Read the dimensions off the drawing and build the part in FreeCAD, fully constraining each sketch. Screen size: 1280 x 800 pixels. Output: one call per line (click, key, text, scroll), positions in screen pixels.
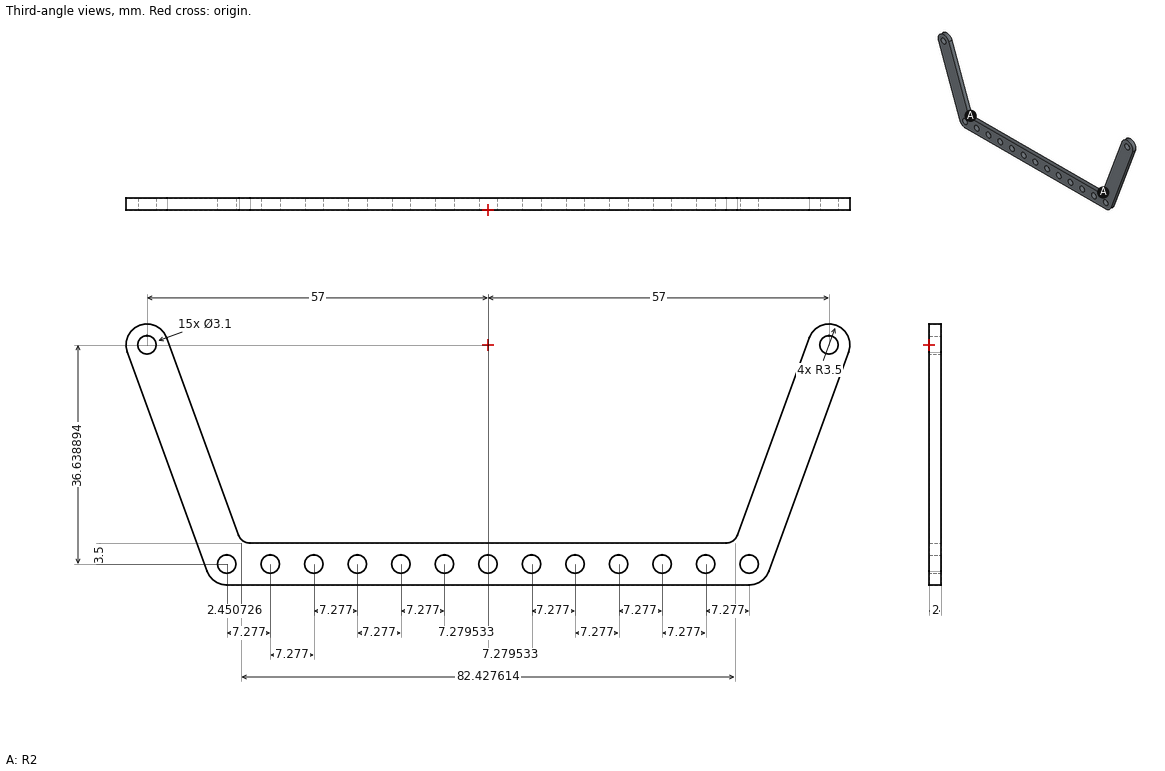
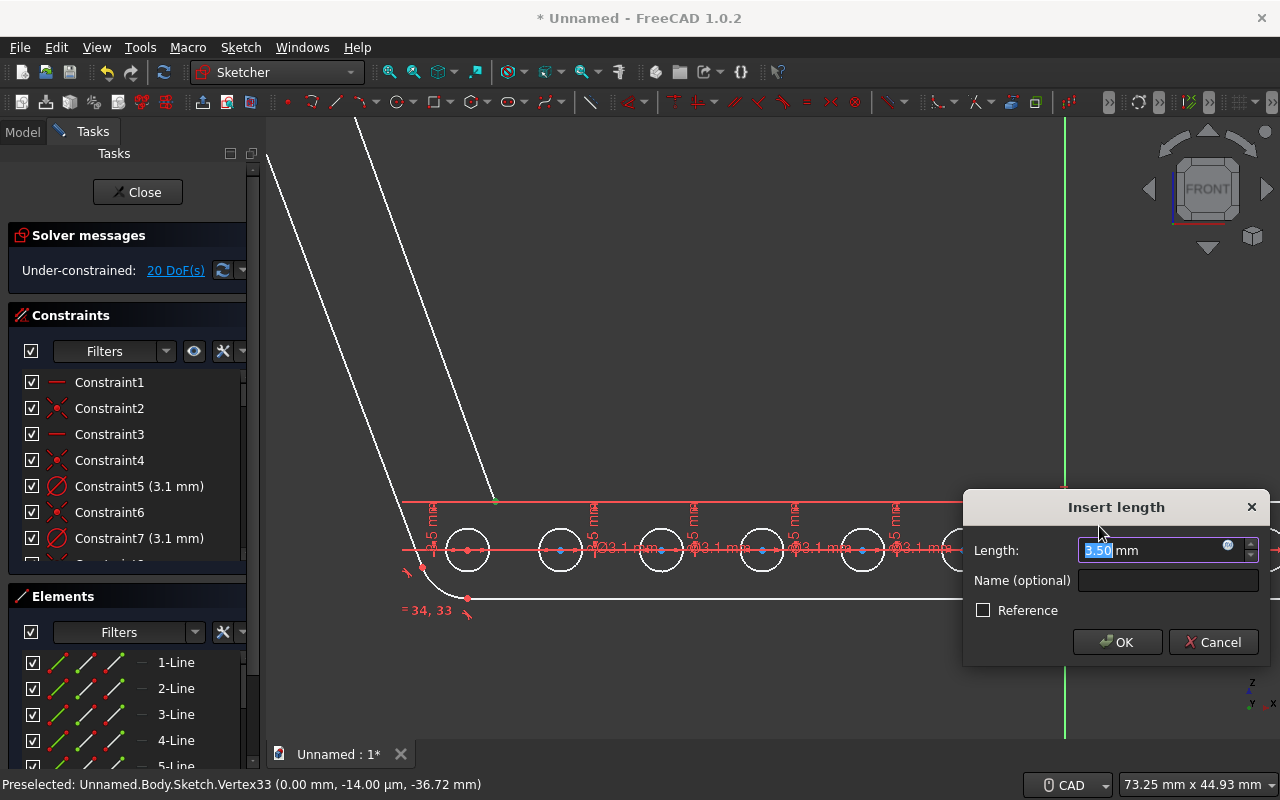
text(3.5)
key(Return)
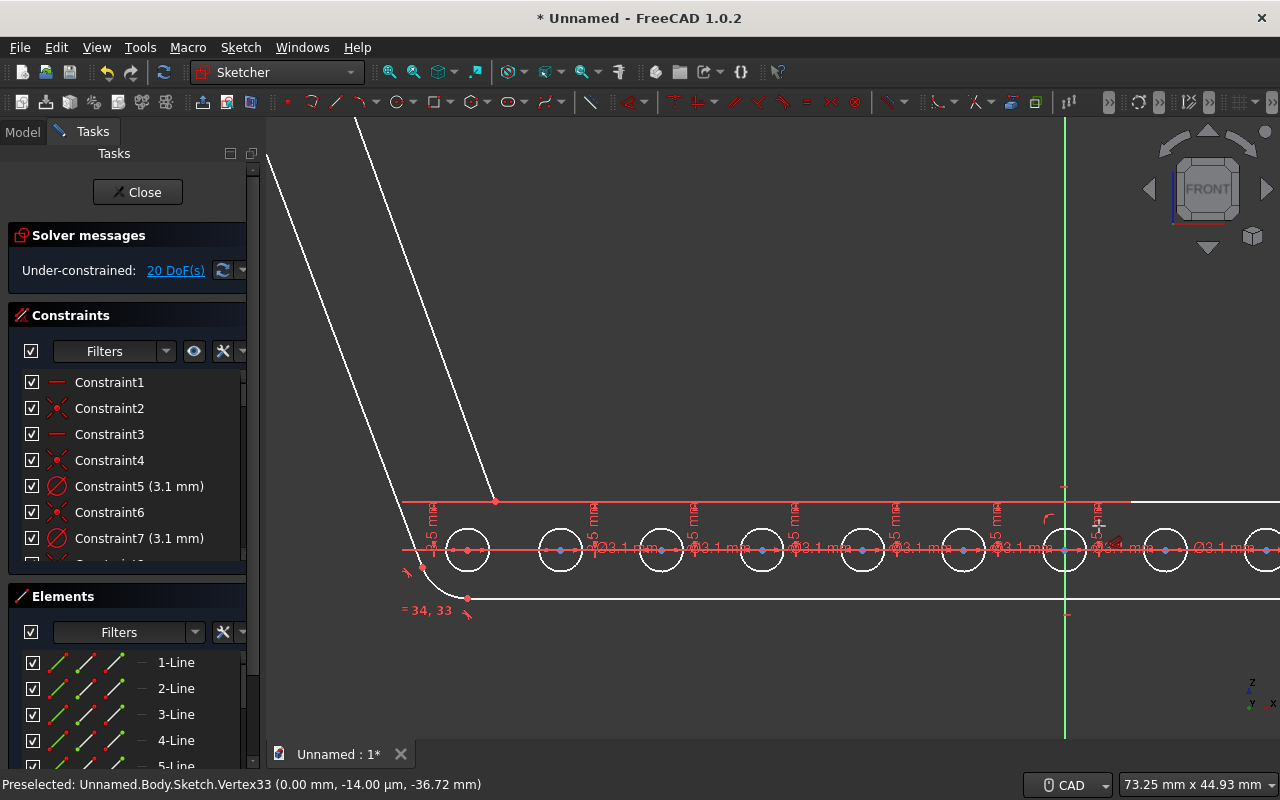
scroll(495, 504, down, 5)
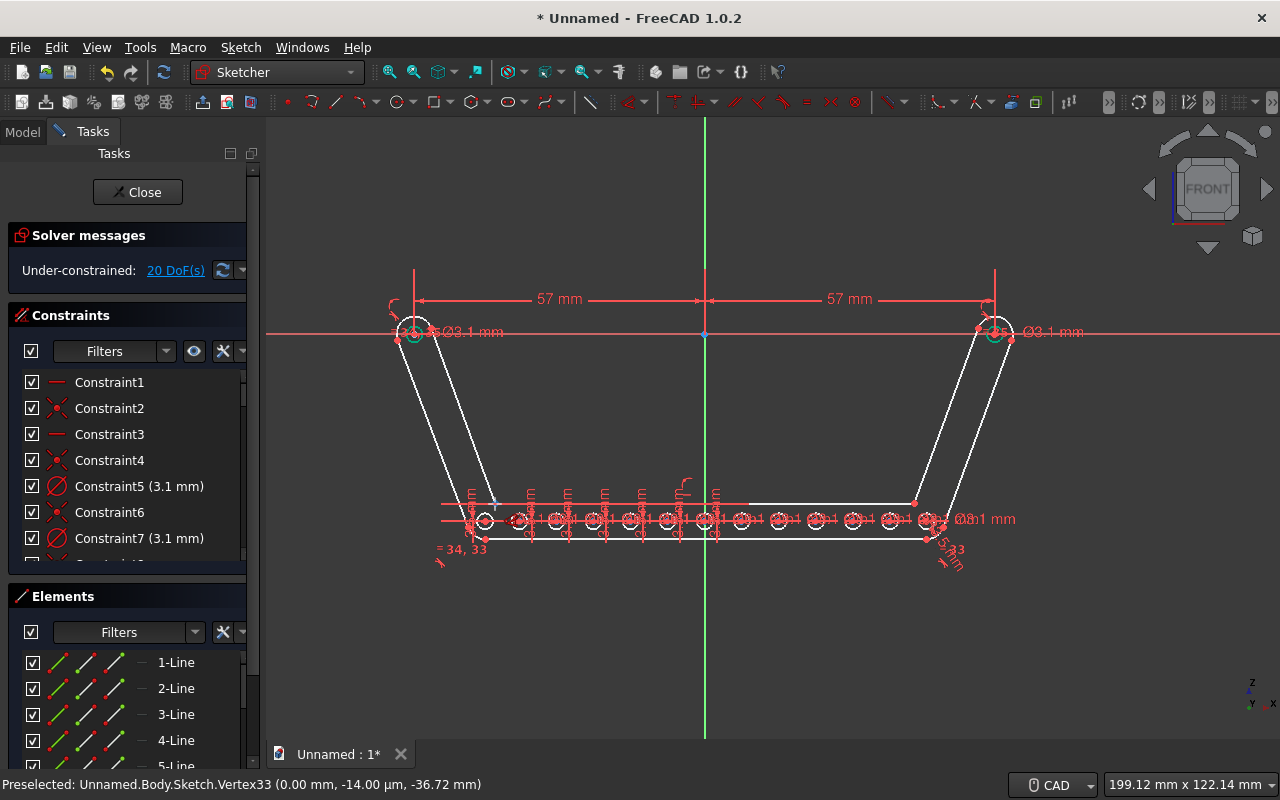
scroll(914, 504, up, 5)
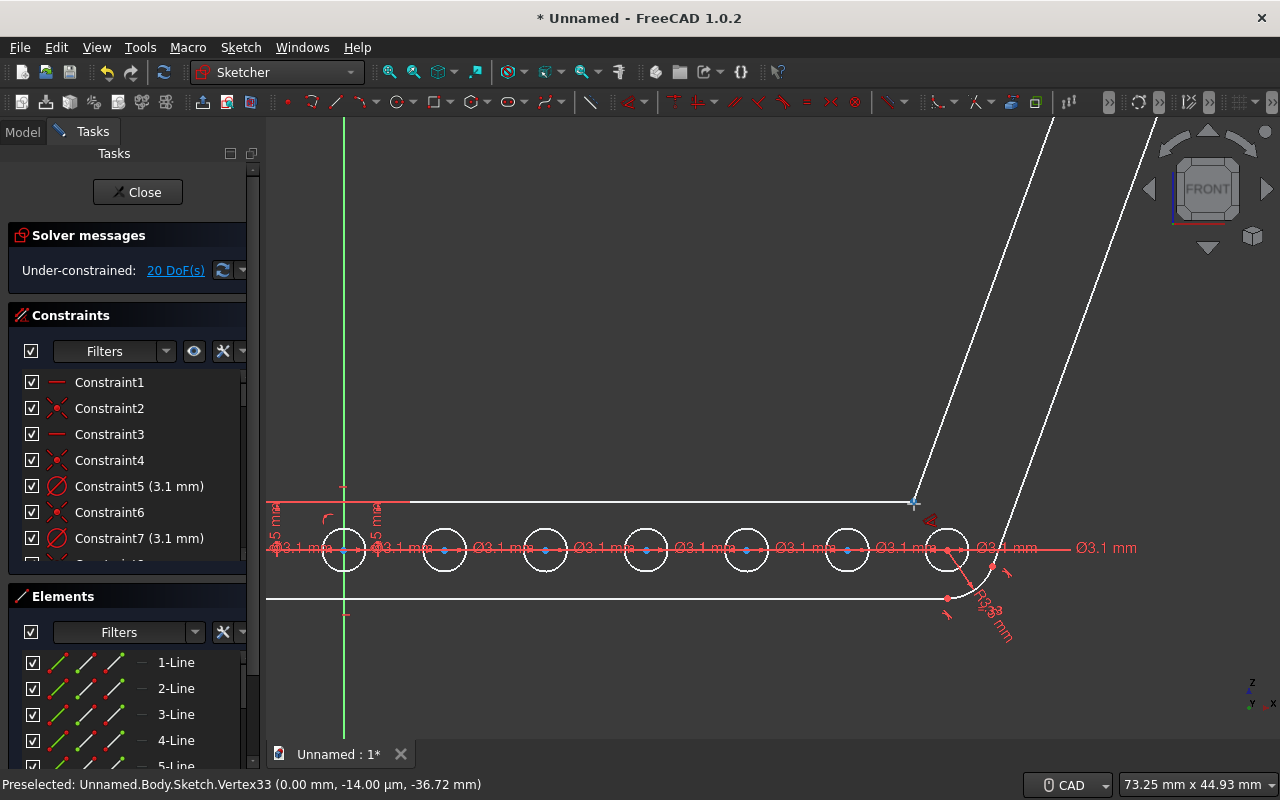
click(913, 502)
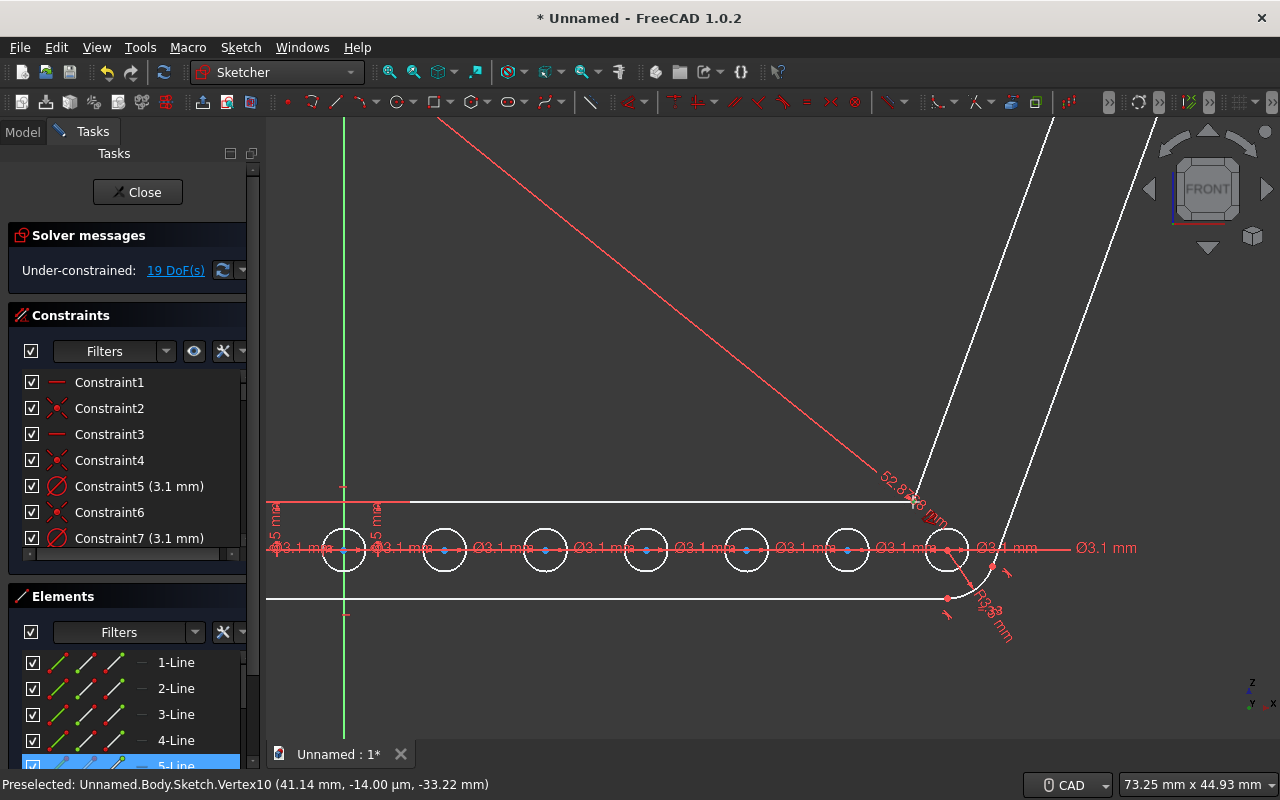
click(445, 550)
click(947, 515)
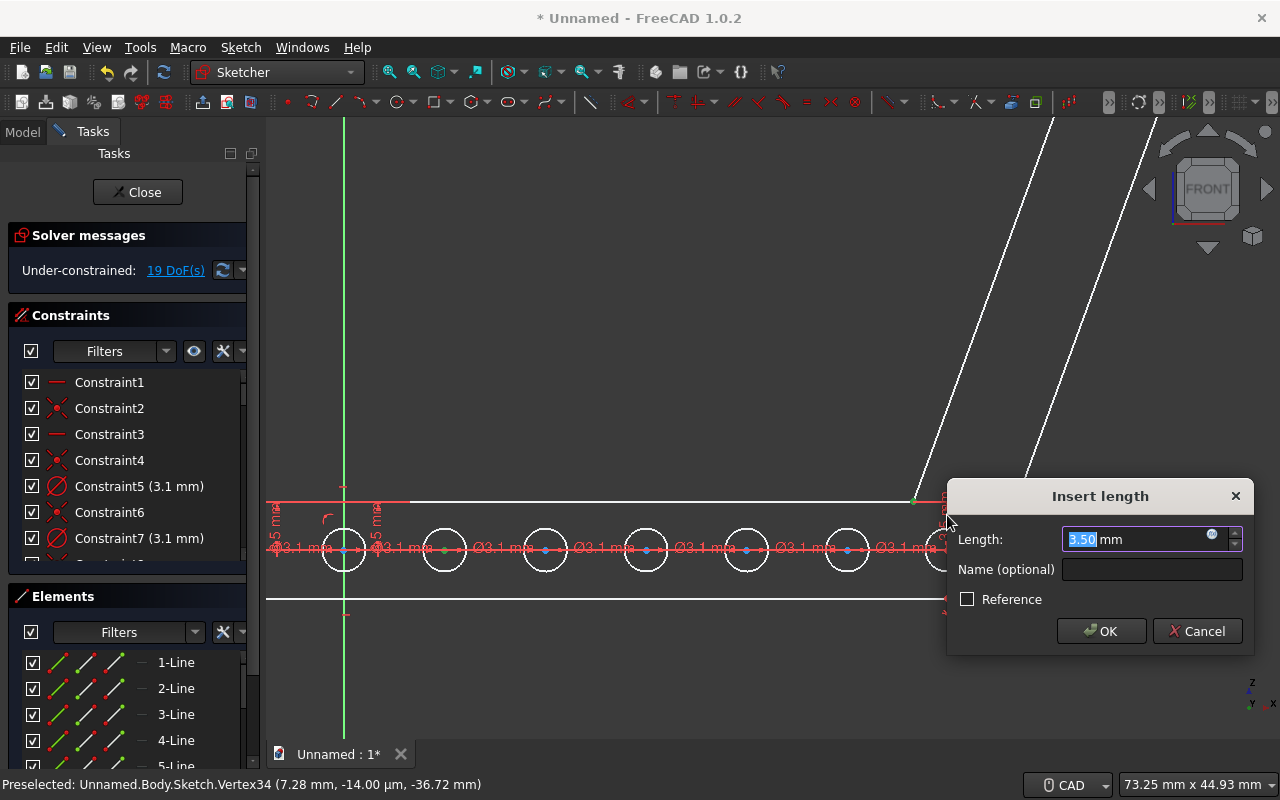
text(3.5)
key(Return)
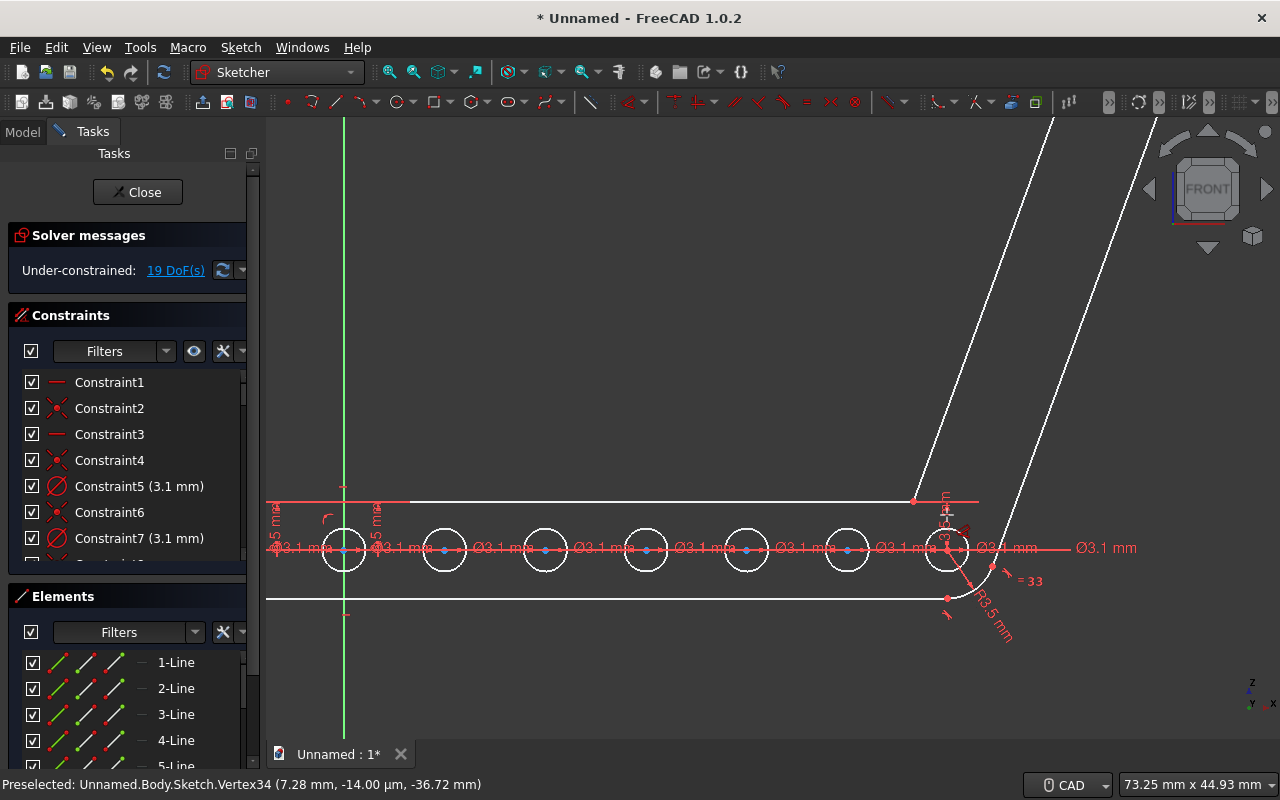
click(913, 502)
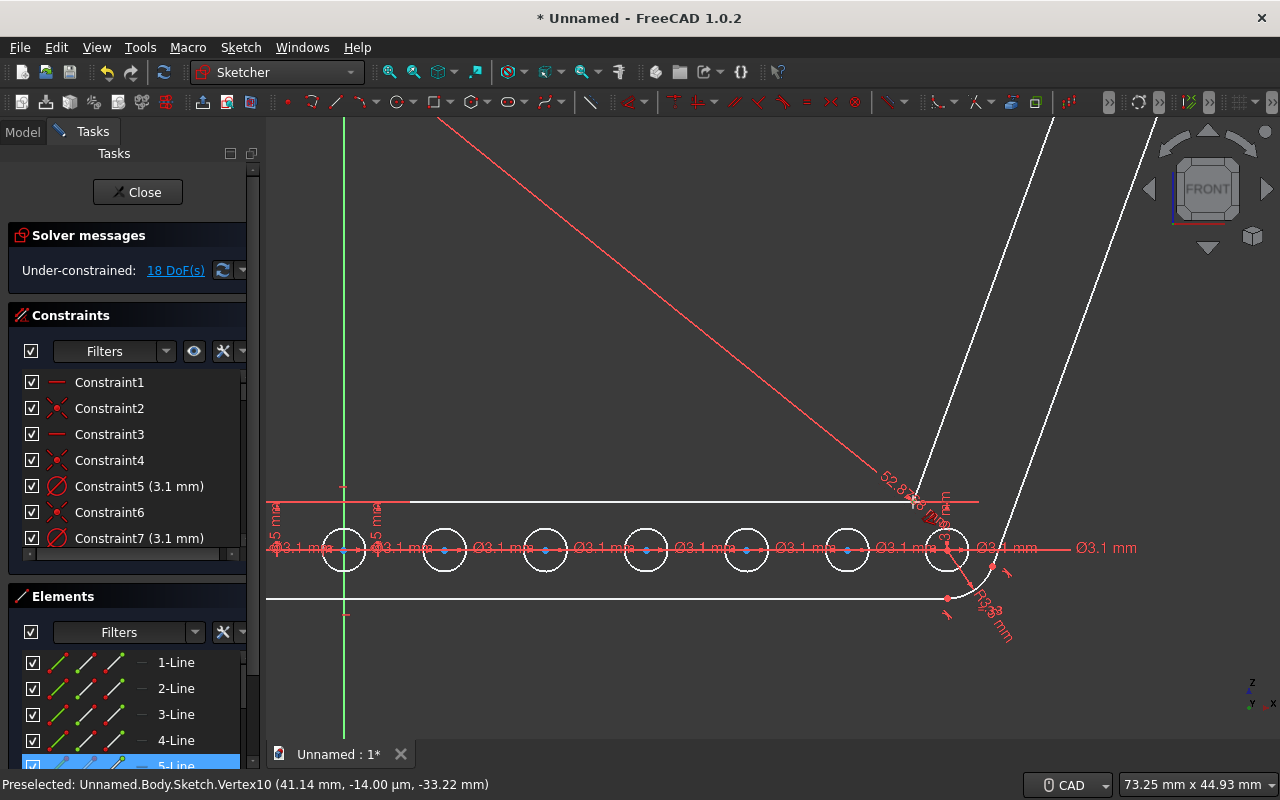
click(545, 550)
click(947, 543)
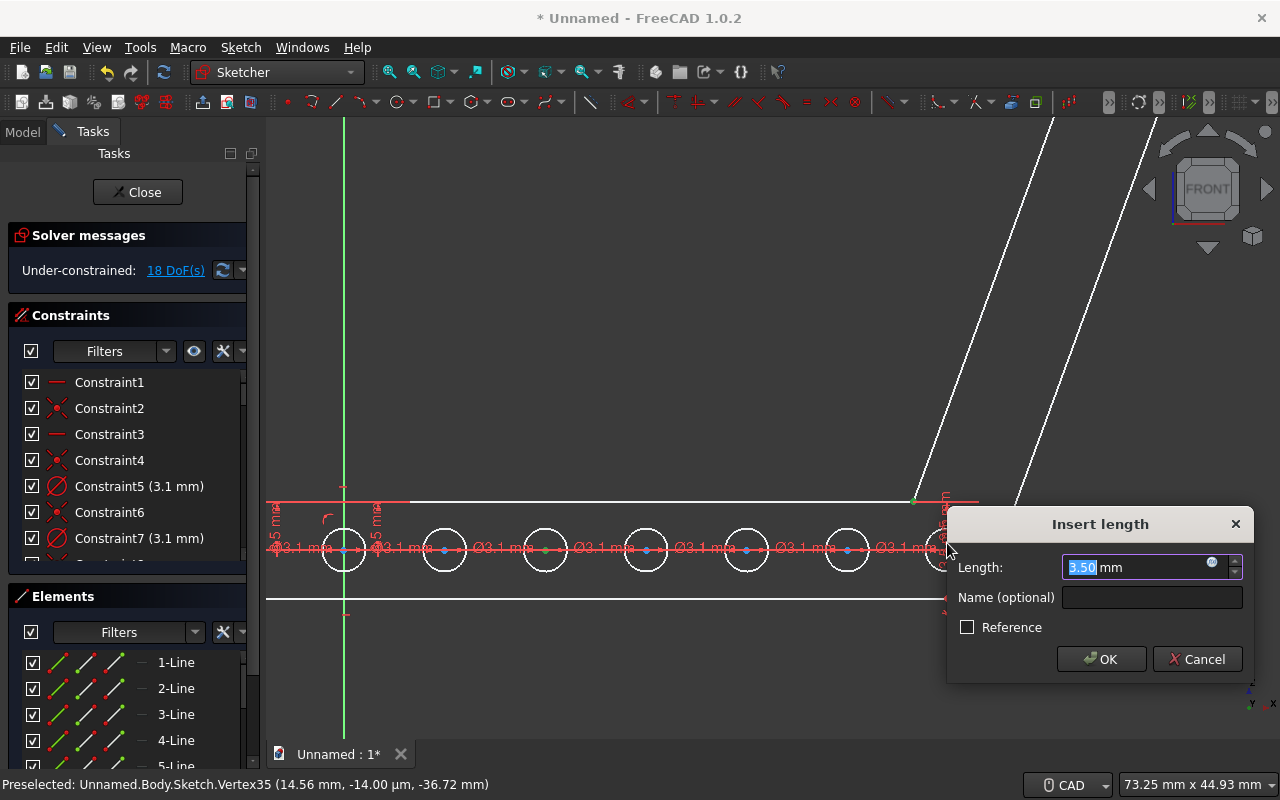
text(3.5)
key(Return)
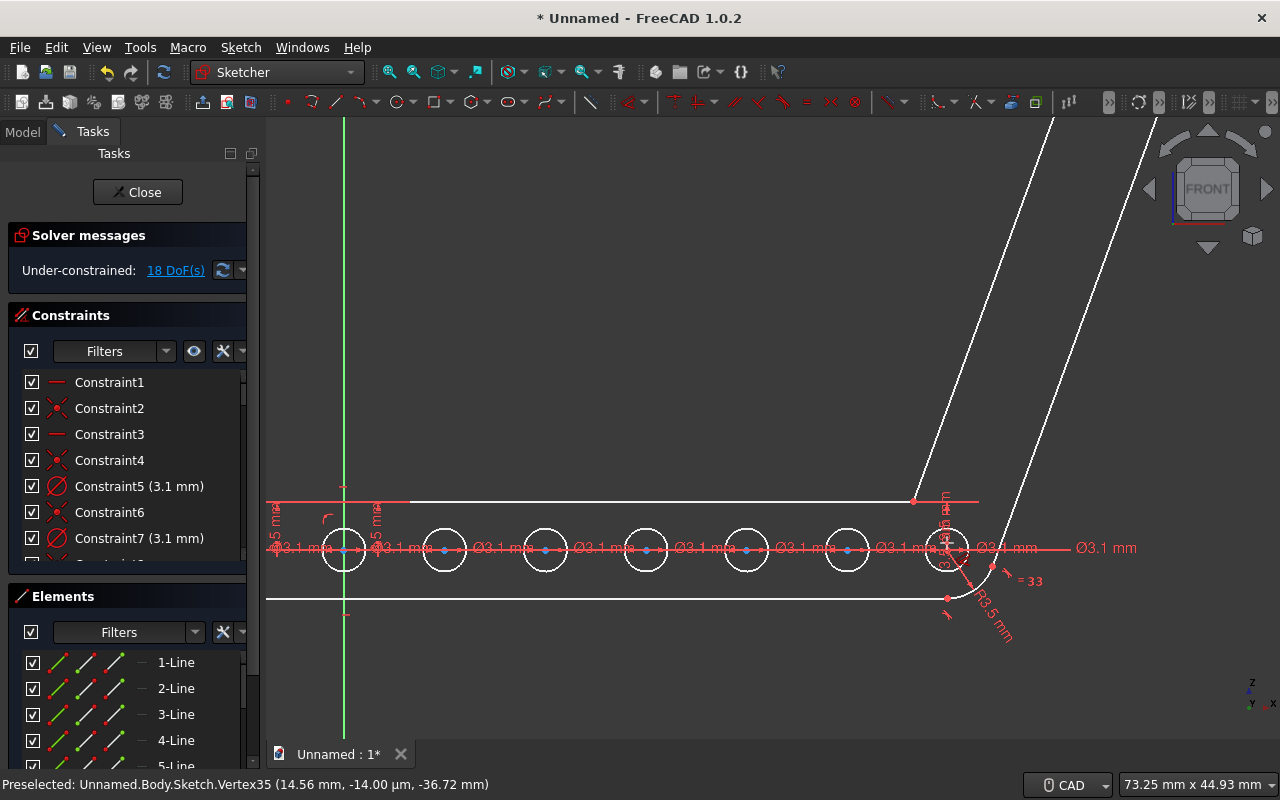
click(913, 502)